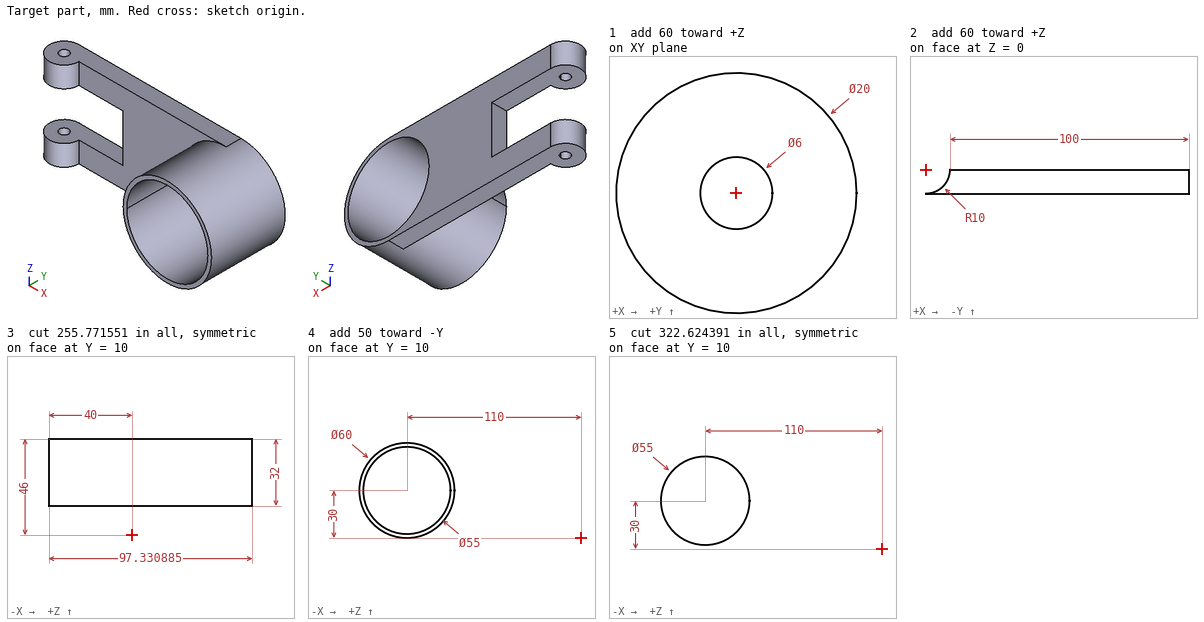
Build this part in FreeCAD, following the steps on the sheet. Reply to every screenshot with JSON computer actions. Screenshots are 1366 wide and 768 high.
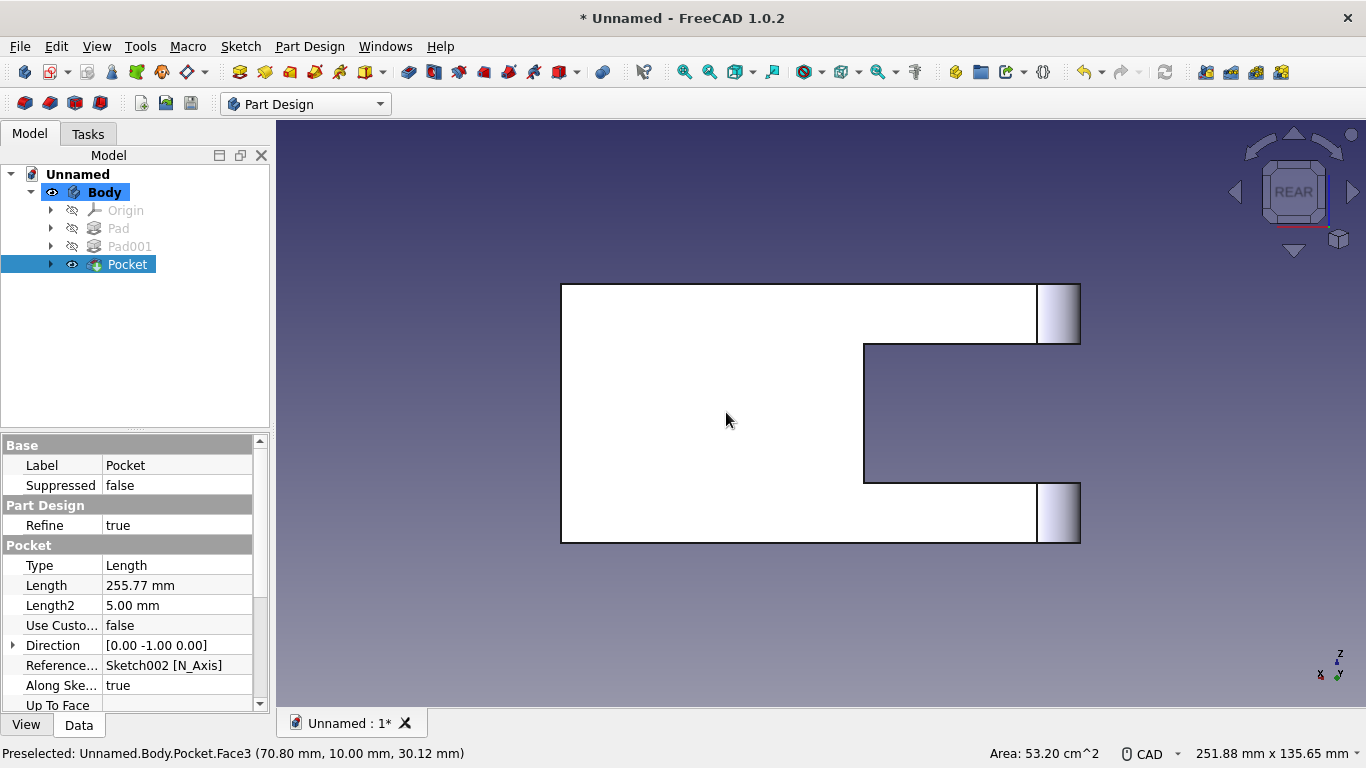
{"action": "left_click", "coordinate": [50, 72]}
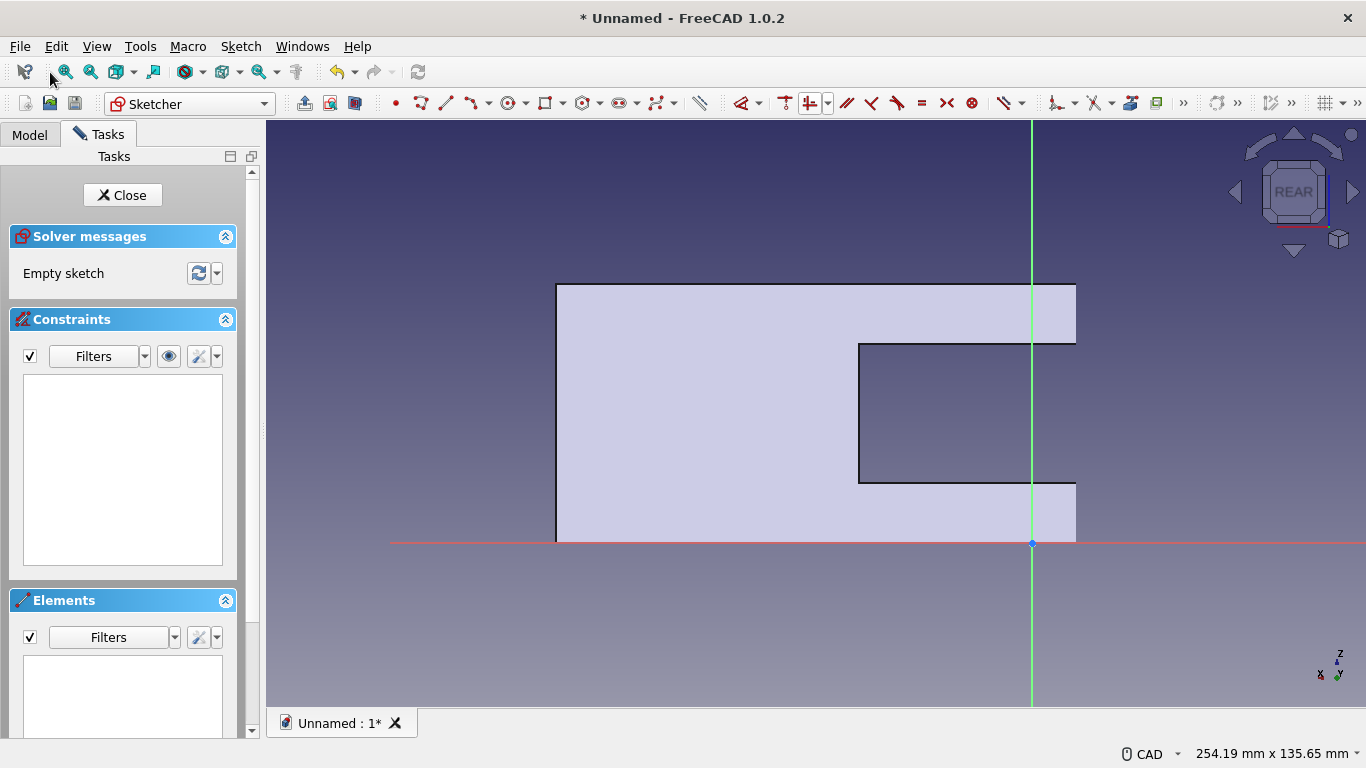
{"action": "left_click", "coordinate": [508, 104]}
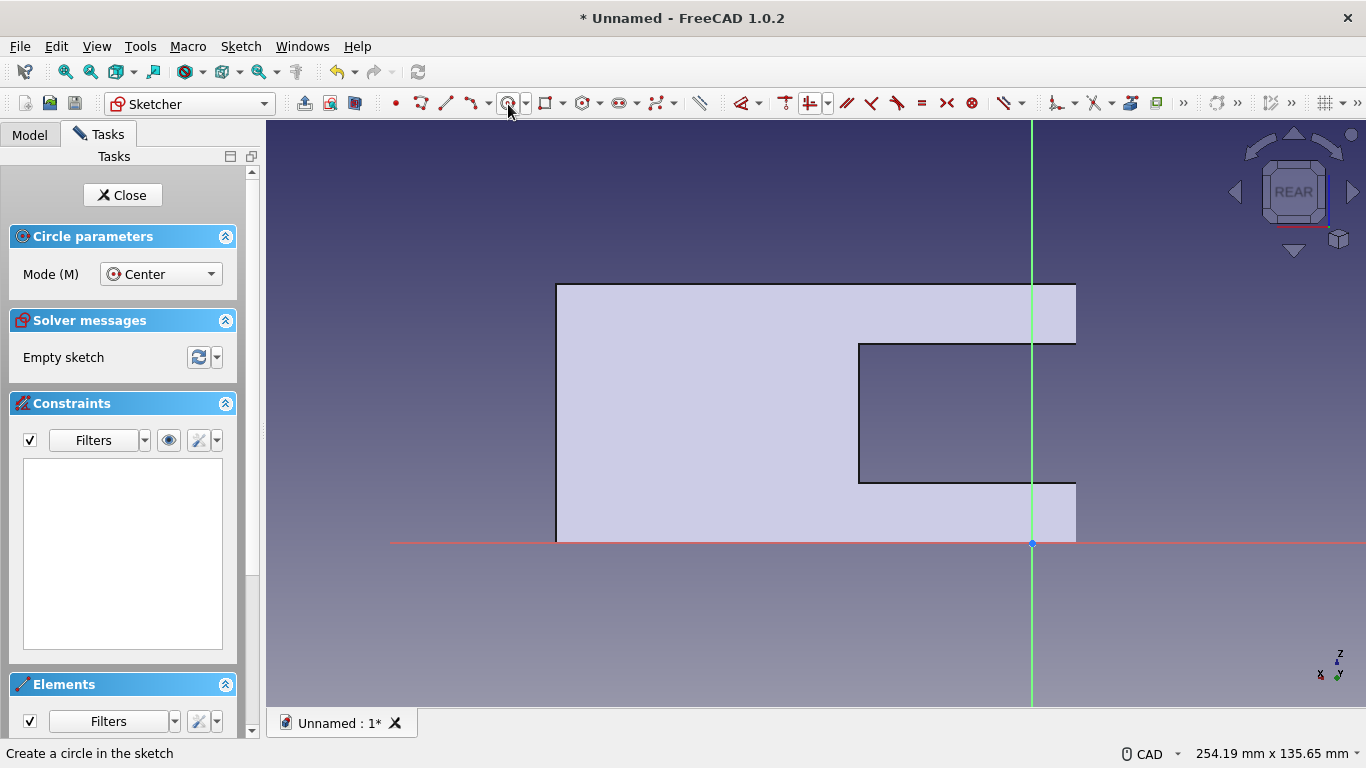
{"action": "left_click", "coordinate": [556, 414]}
{"action": "mouse_move", "coordinate": [648, 322]}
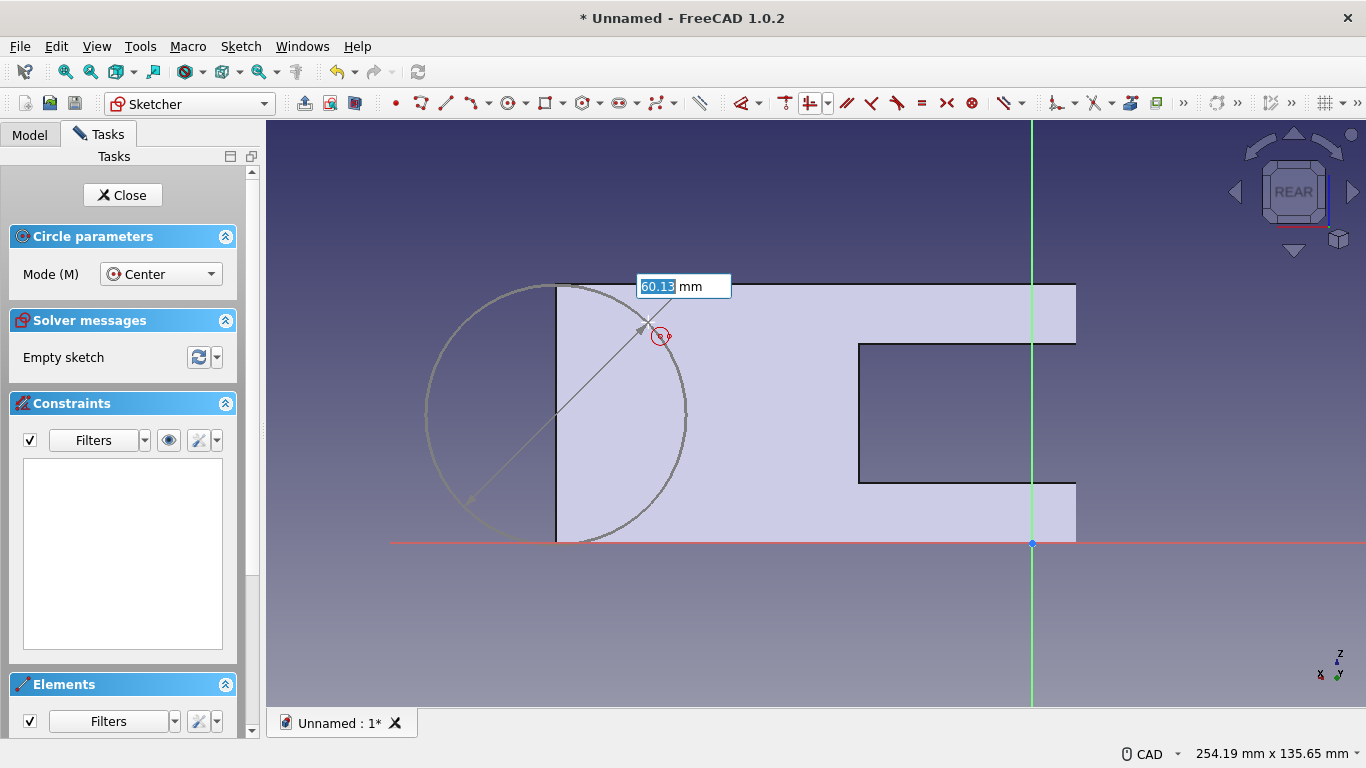
{"action": "type", "text": "60"}
{"action": "key", "text": "Return"}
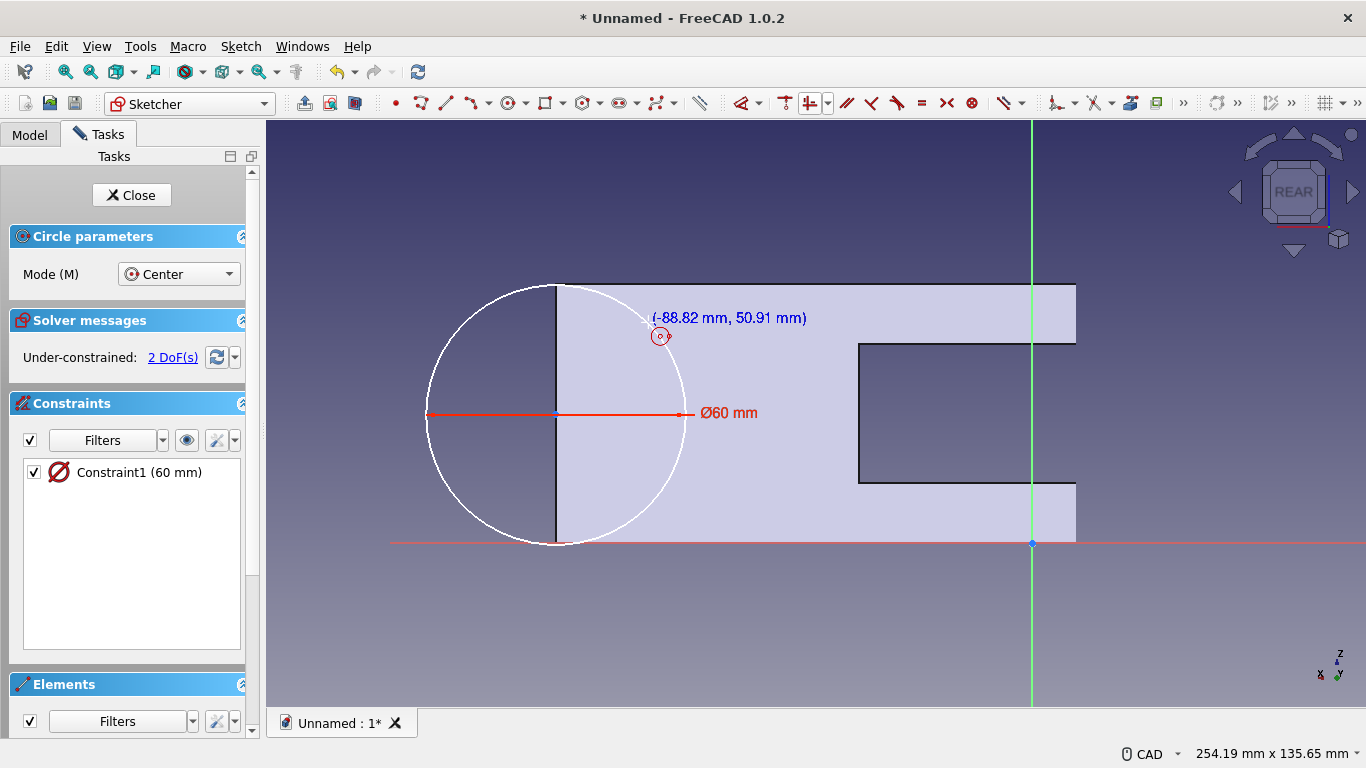
{"action": "left_click", "coordinate": [556, 415]}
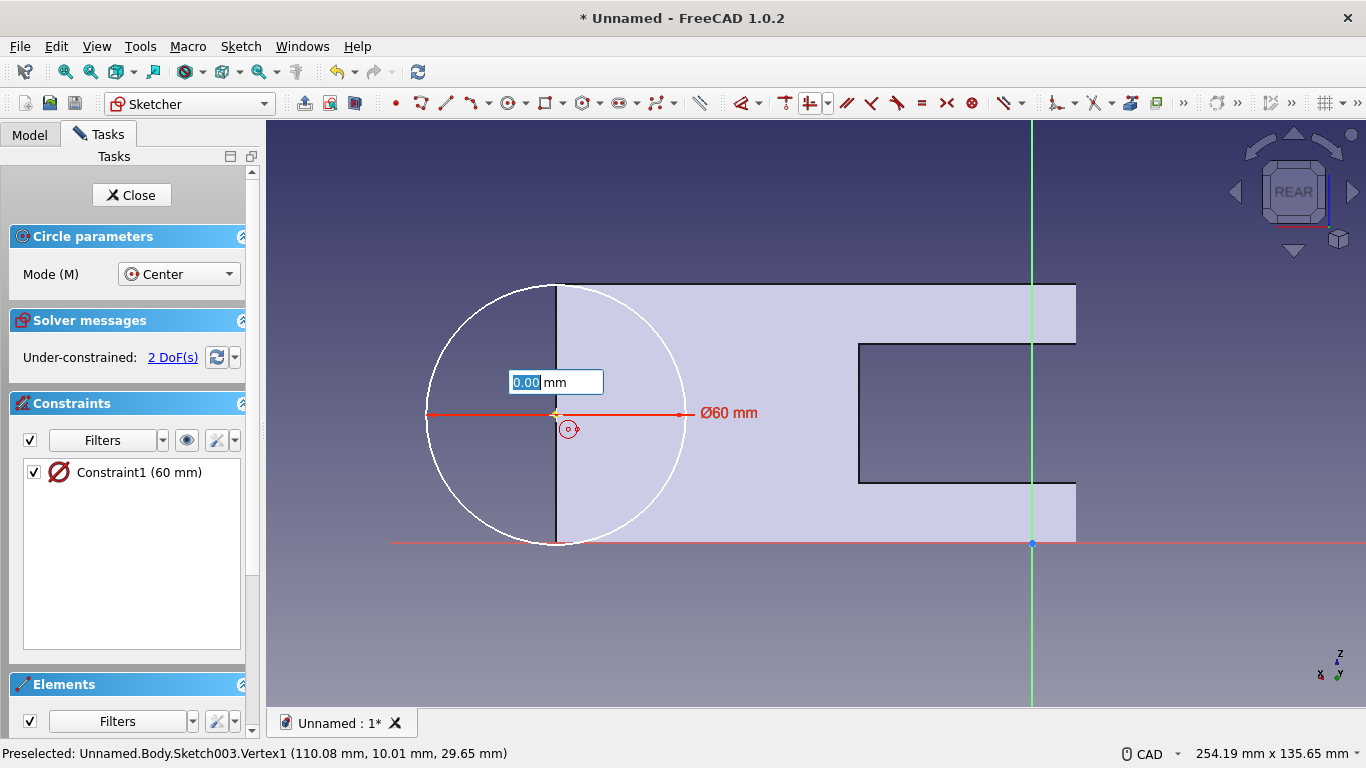
{"action": "scroll", "coordinate": [472, 329], "scroll_direction": "up", "scroll_amount": 2}
{"action": "mouse_move", "coordinate": [472, 329]}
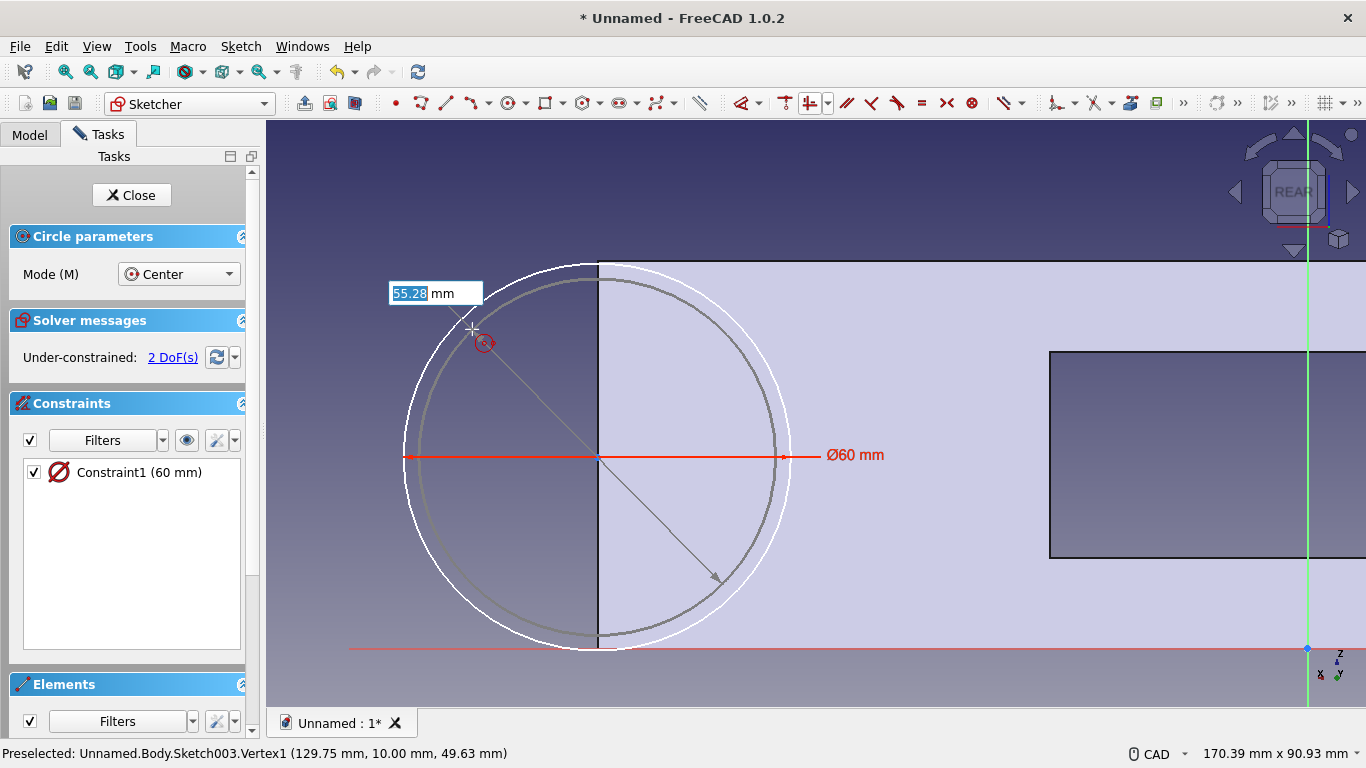
{"action": "type", "text": "55"}
{"action": "key", "text": "Return"}
{"action": "key", "text": "Escape"}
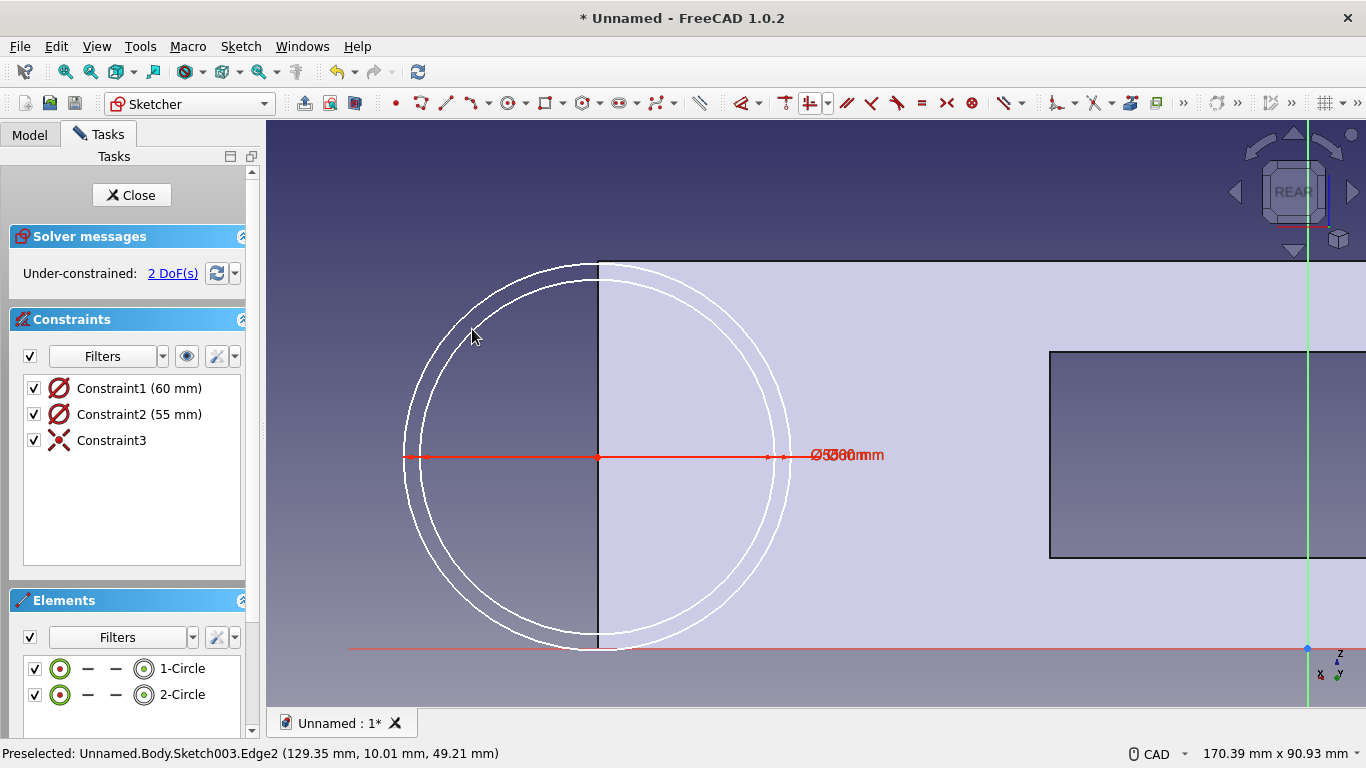
{"action": "left_click", "coordinate": [740, 104]}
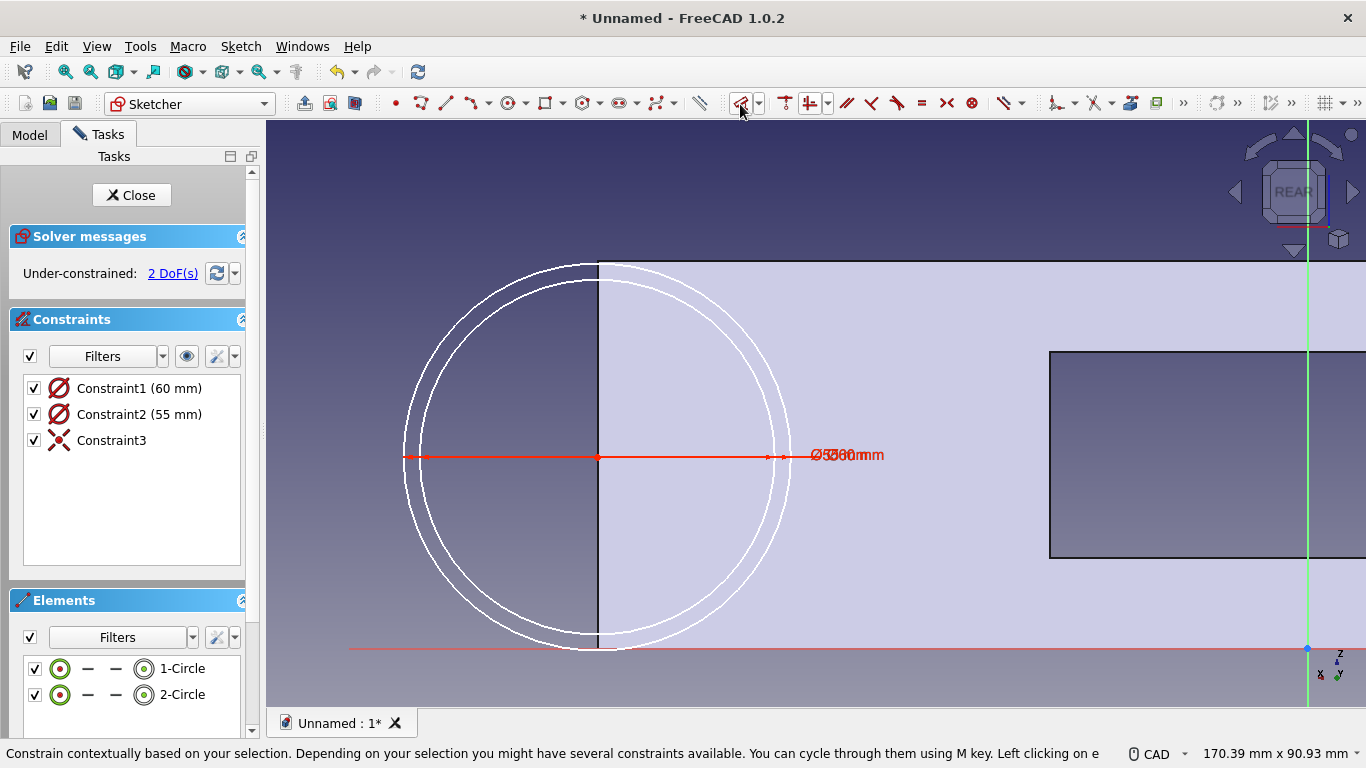
{"action": "left_click", "coordinate": [597, 457]}
{"action": "left_click", "coordinate": [563, 553]}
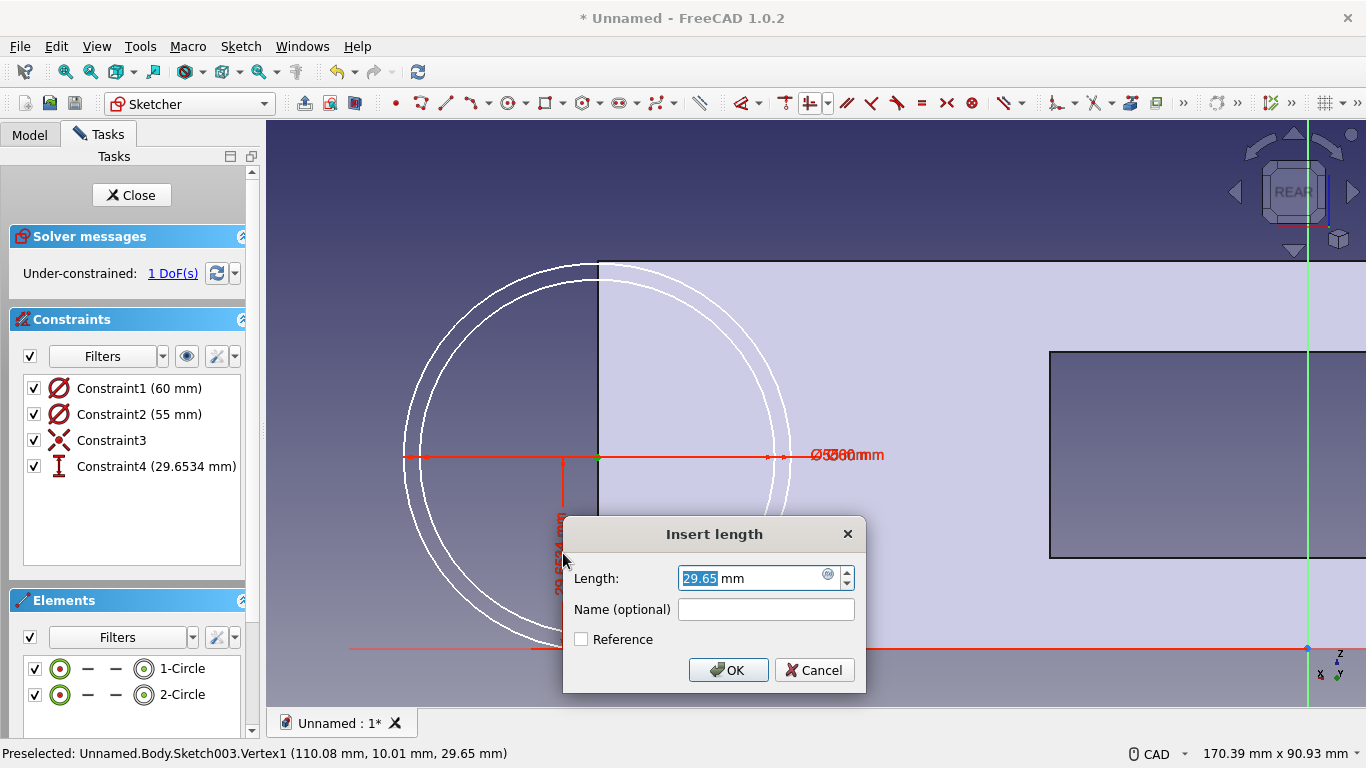
{"action": "type", "text": "30"}
{"action": "key", "text": "Return"}